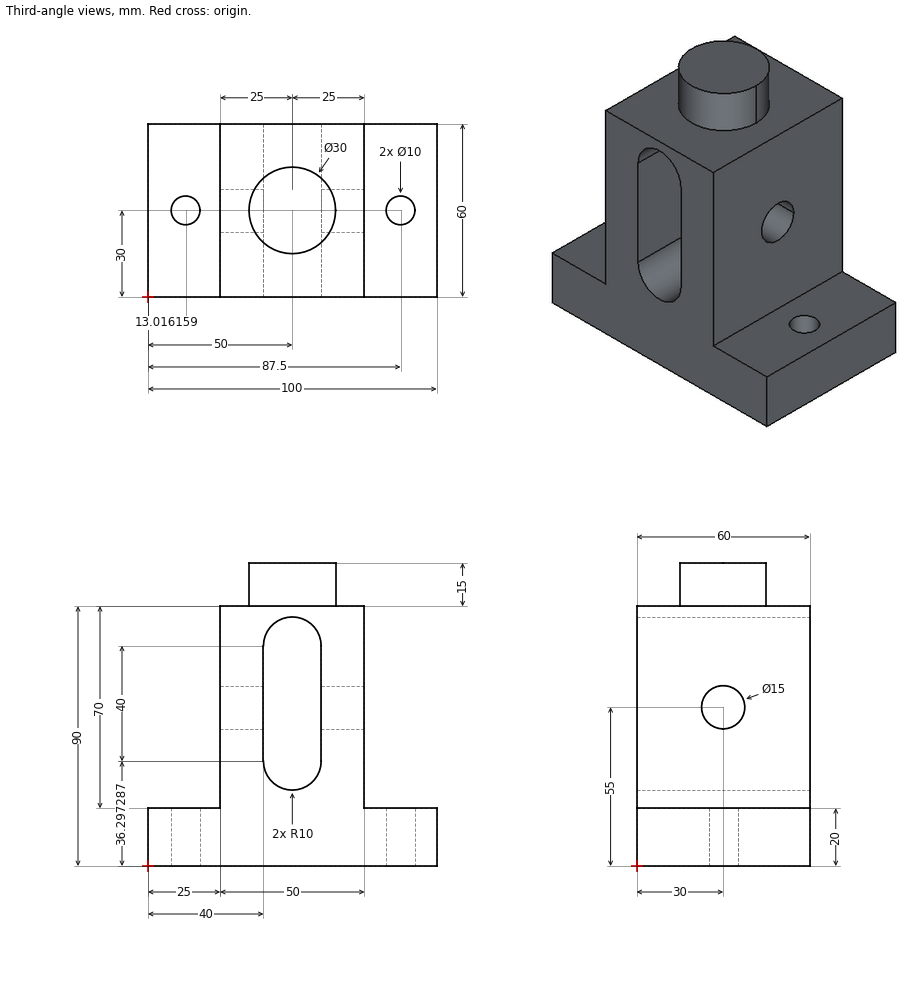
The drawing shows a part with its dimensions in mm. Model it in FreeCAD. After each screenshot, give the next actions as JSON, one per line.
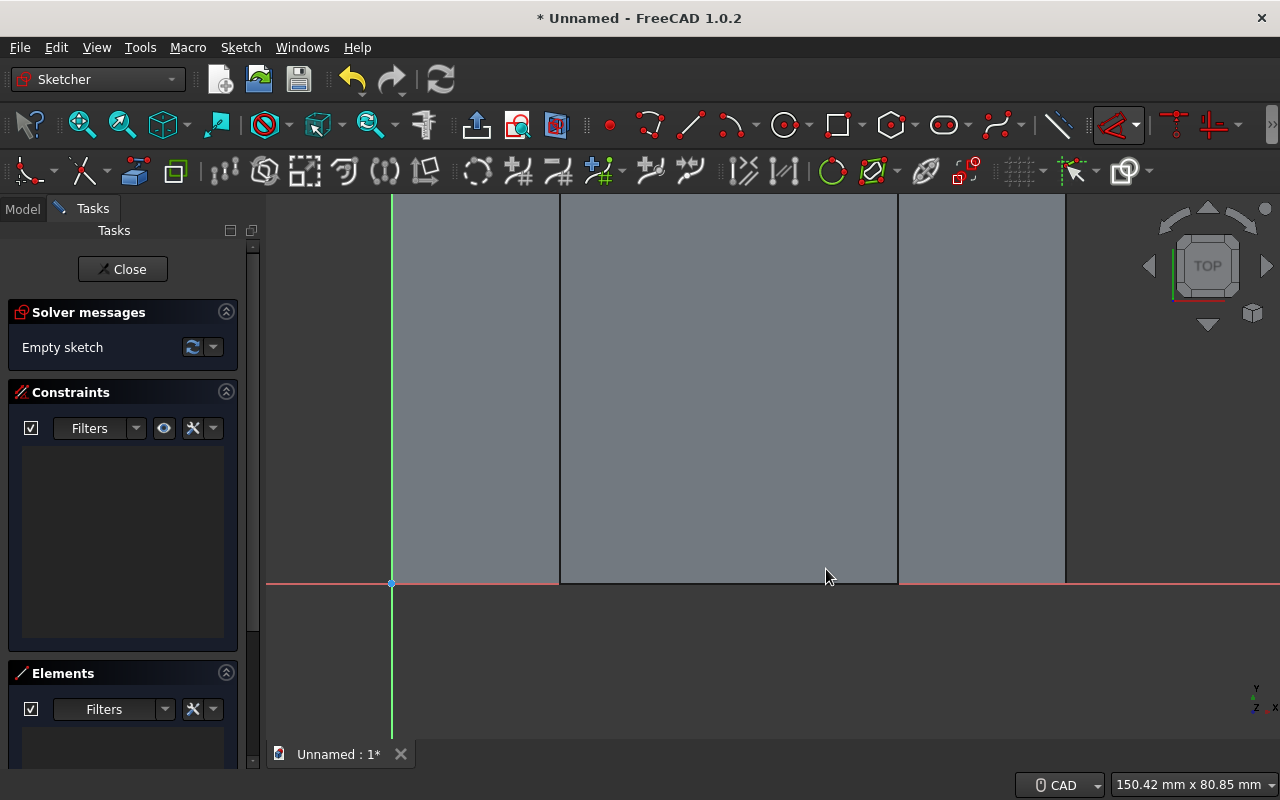
{"action": "left_click", "coordinate": [786, 126]}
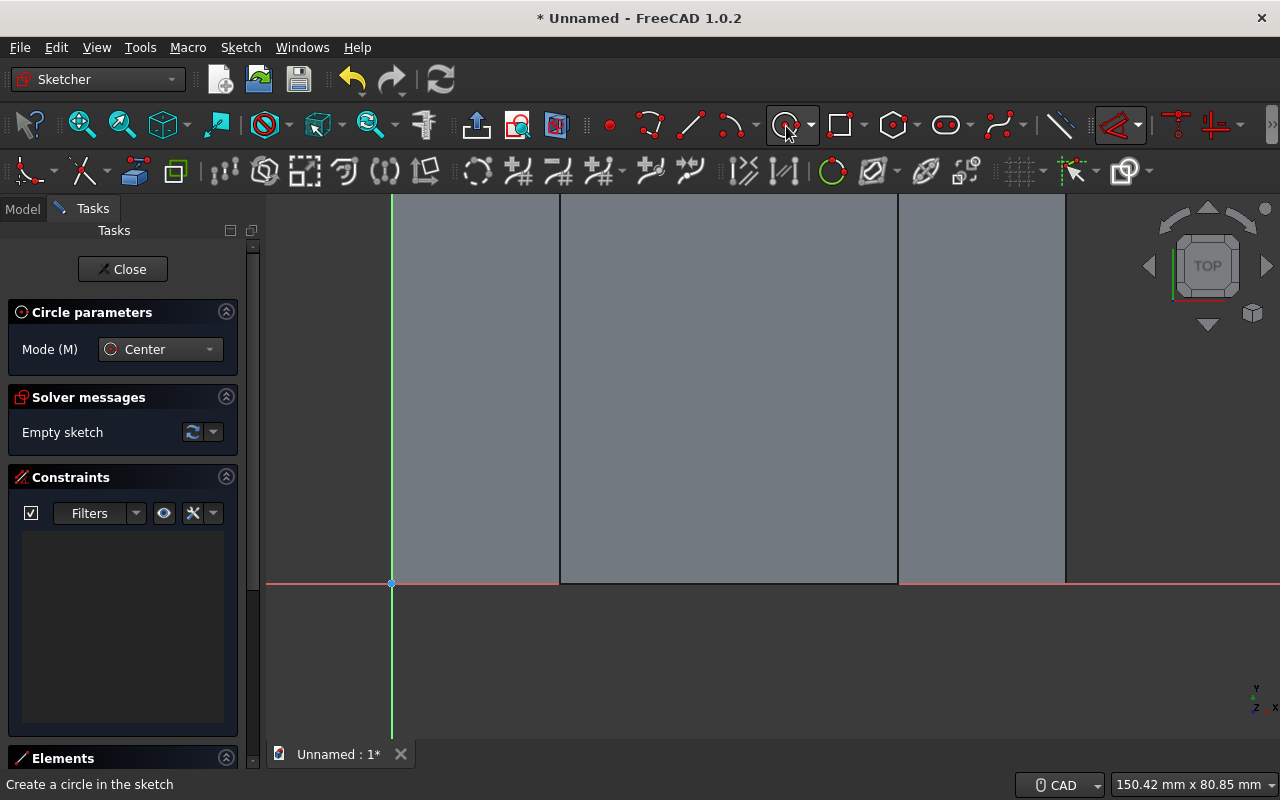
{"action": "left_click", "coordinate": [982, 382]}
{"action": "left_click", "coordinate": [1006, 358]}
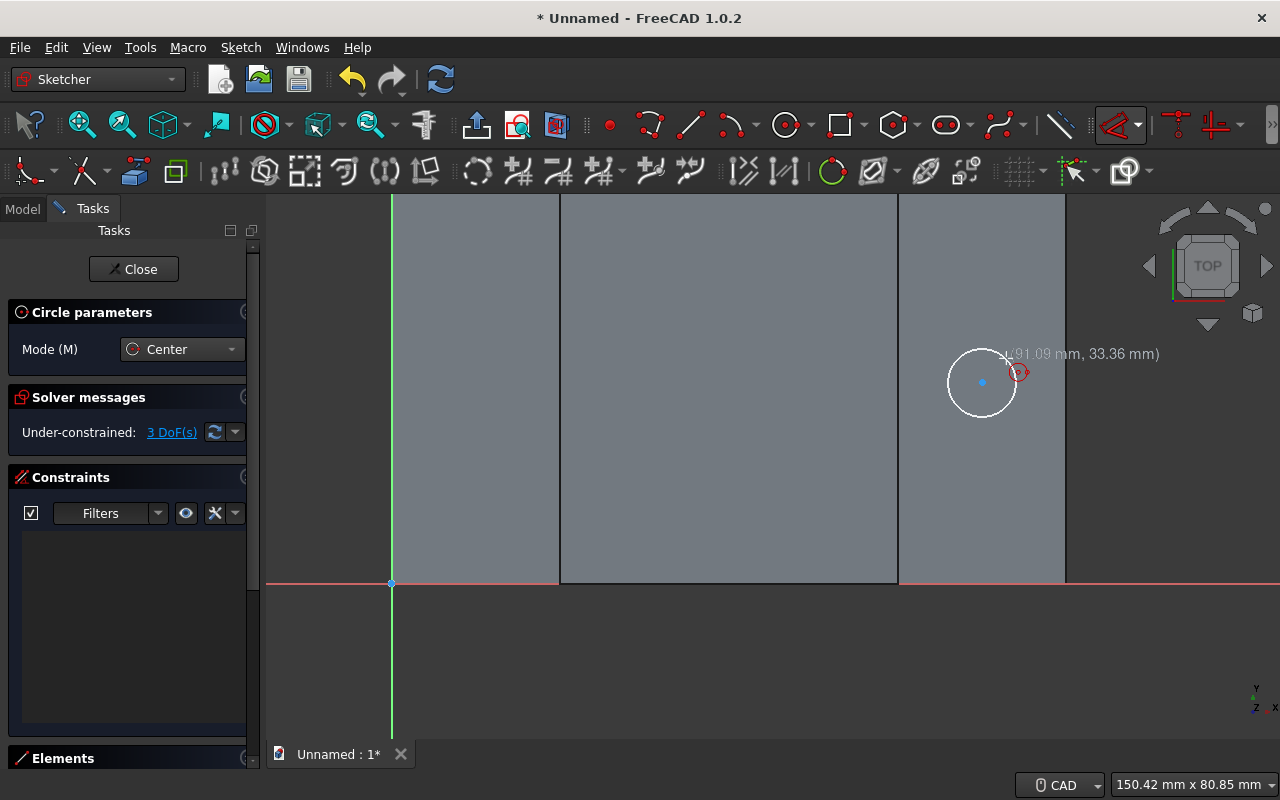
{"action": "left_click", "coordinate": [480, 382]}
{"action": "left_click", "coordinate": [503, 358]}
{"action": "key", "text": "Escape"}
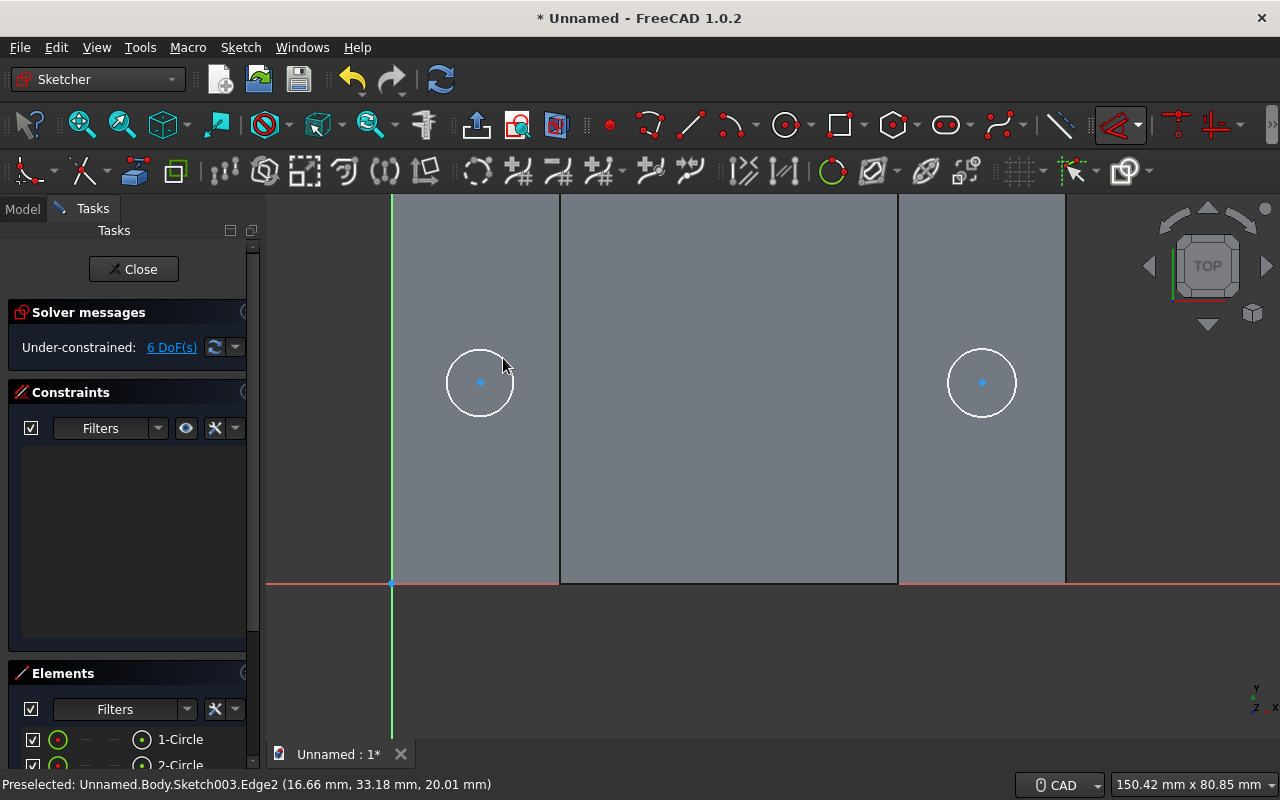
{"action": "left_click", "coordinate": [1006, 359]}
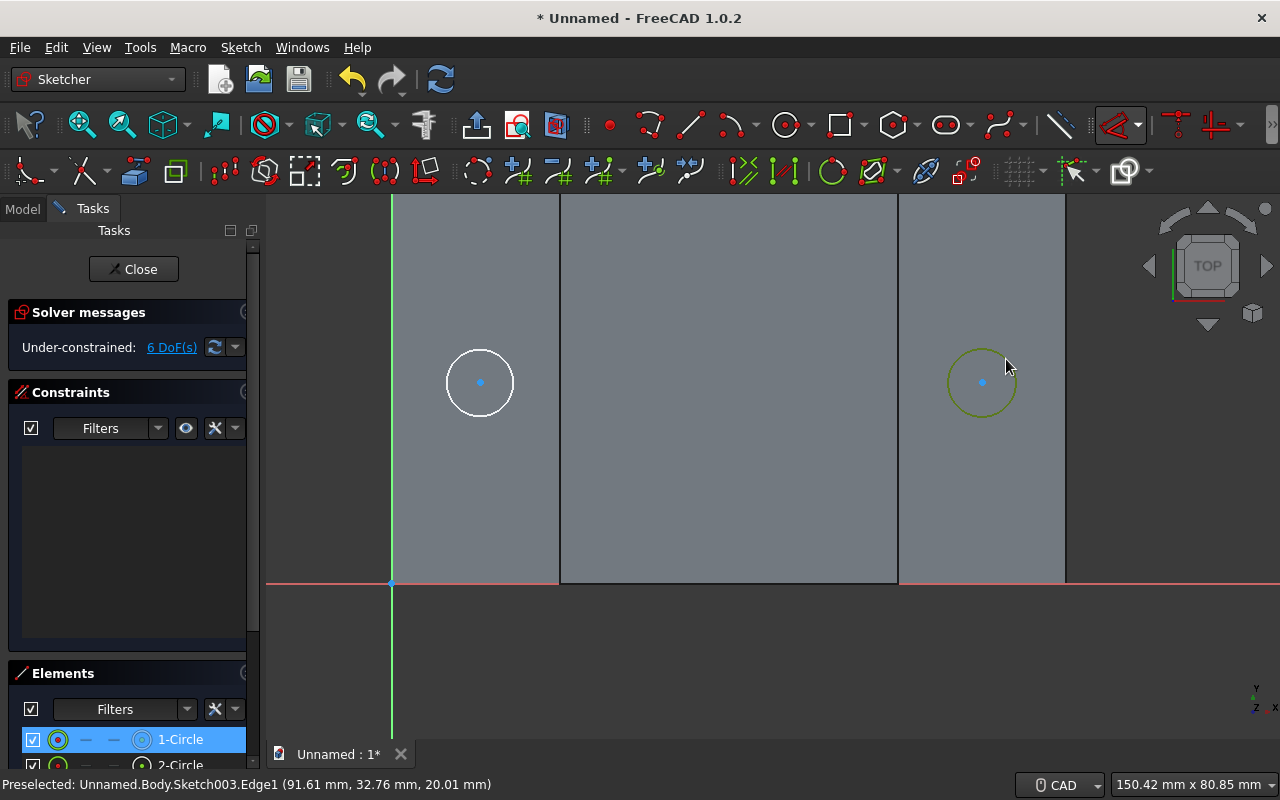
{"action": "left_click", "coordinate": [503, 359]}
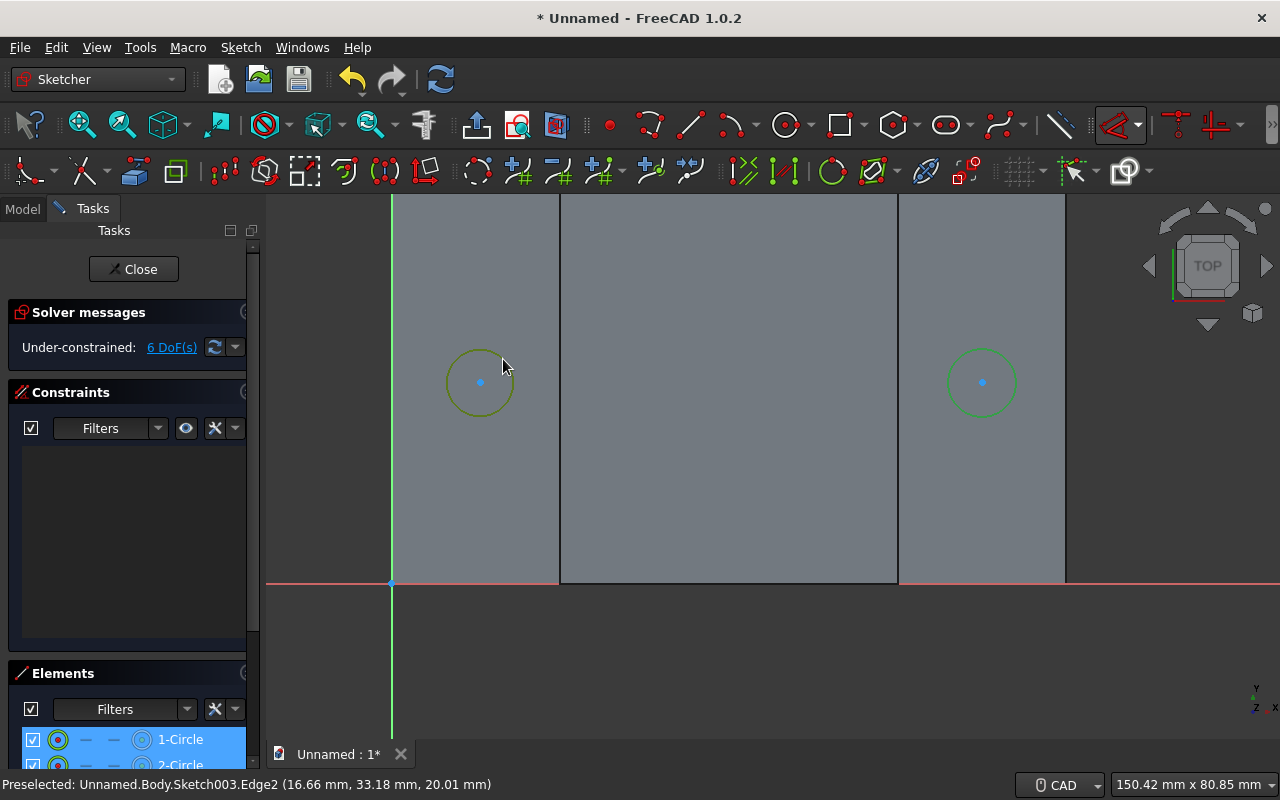
{"action": "key", "text": "e"}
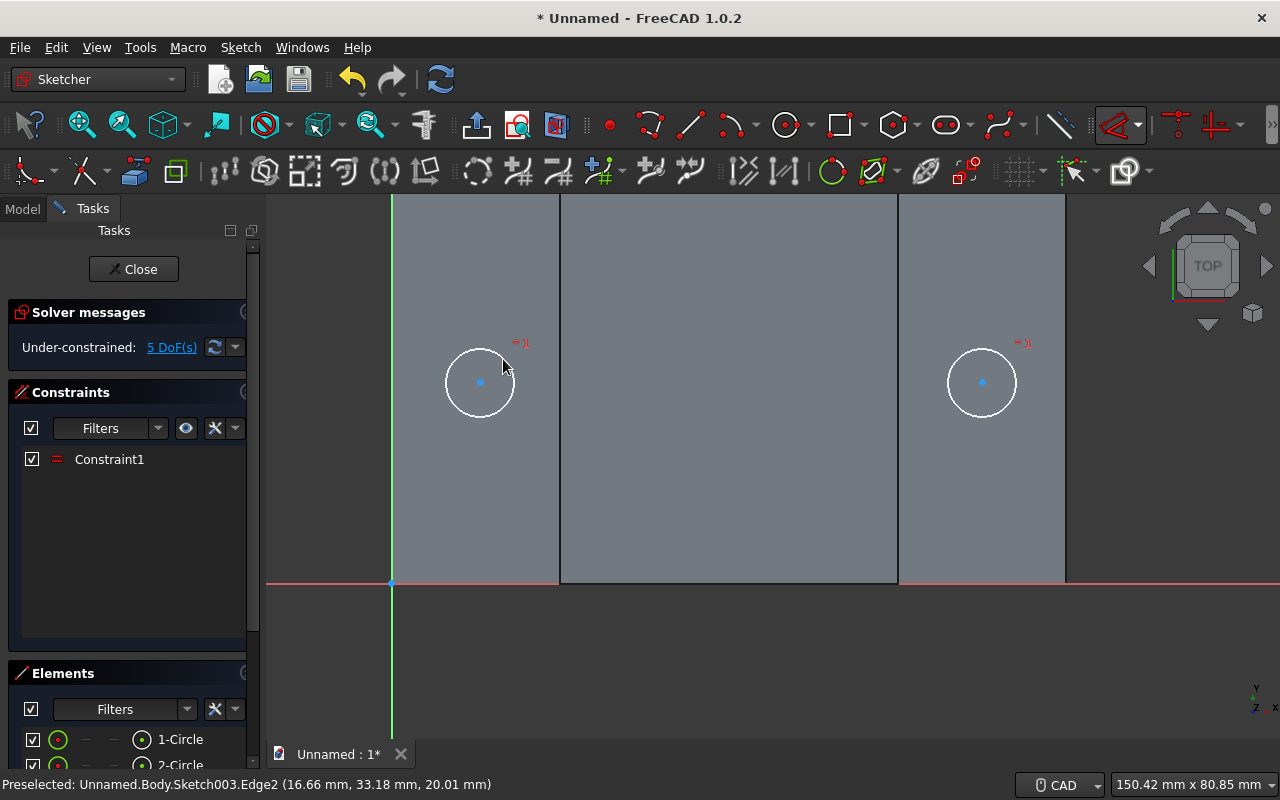
{"action": "left_click", "coordinate": [982, 383]}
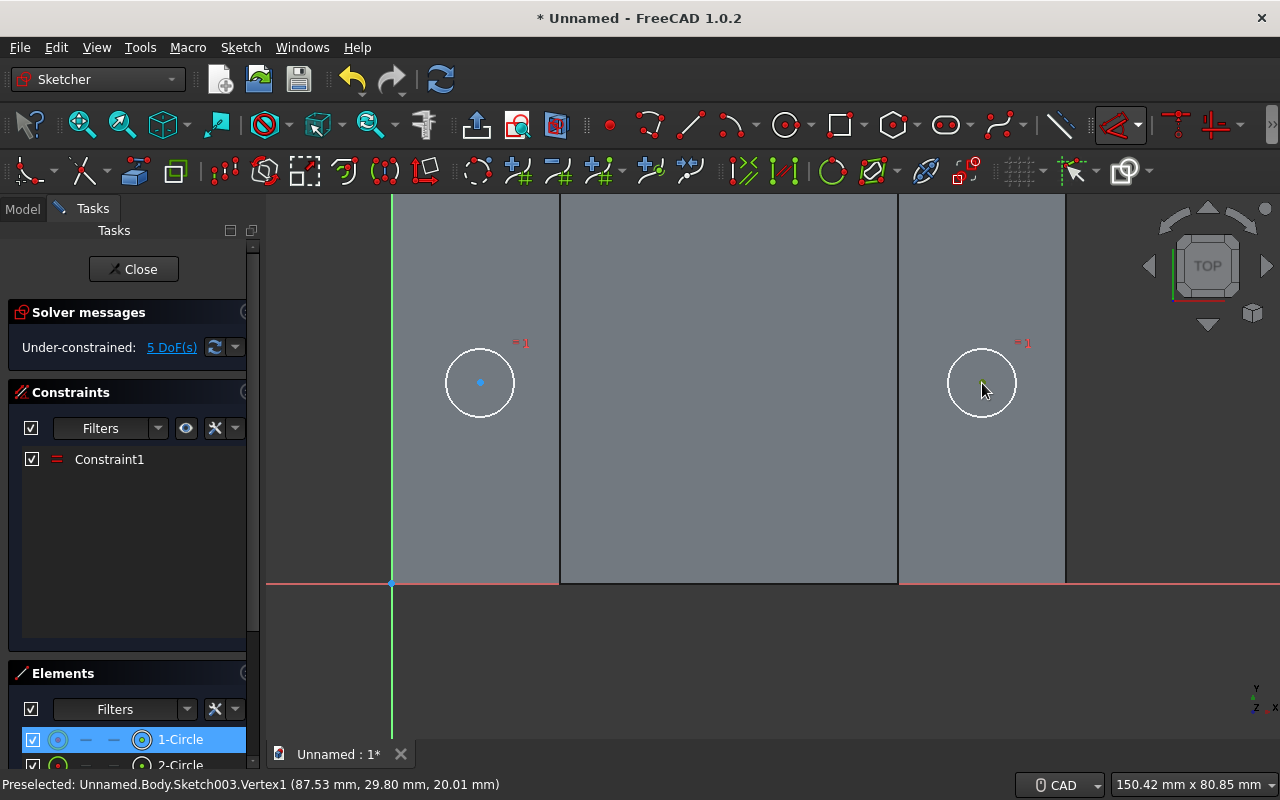
{"action": "left_click", "coordinate": [480, 383]}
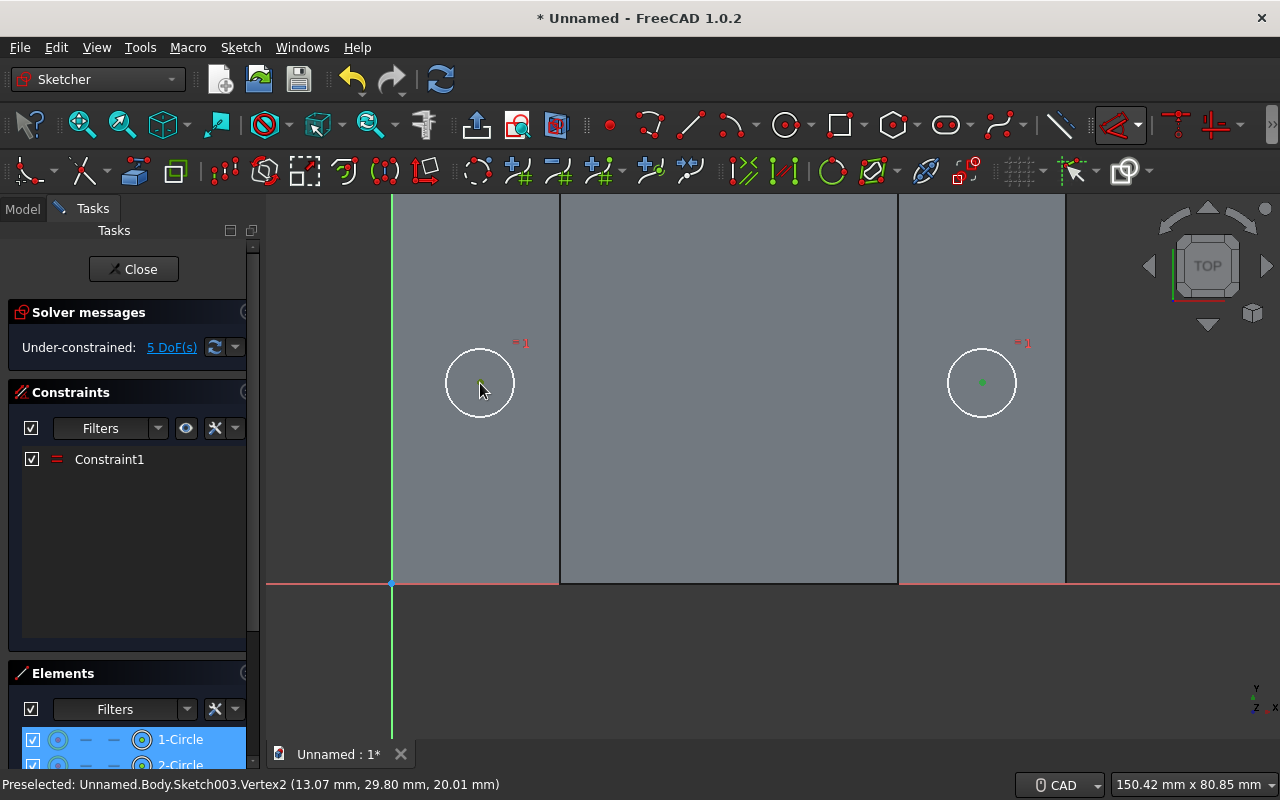
{"action": "key", "text": "h"}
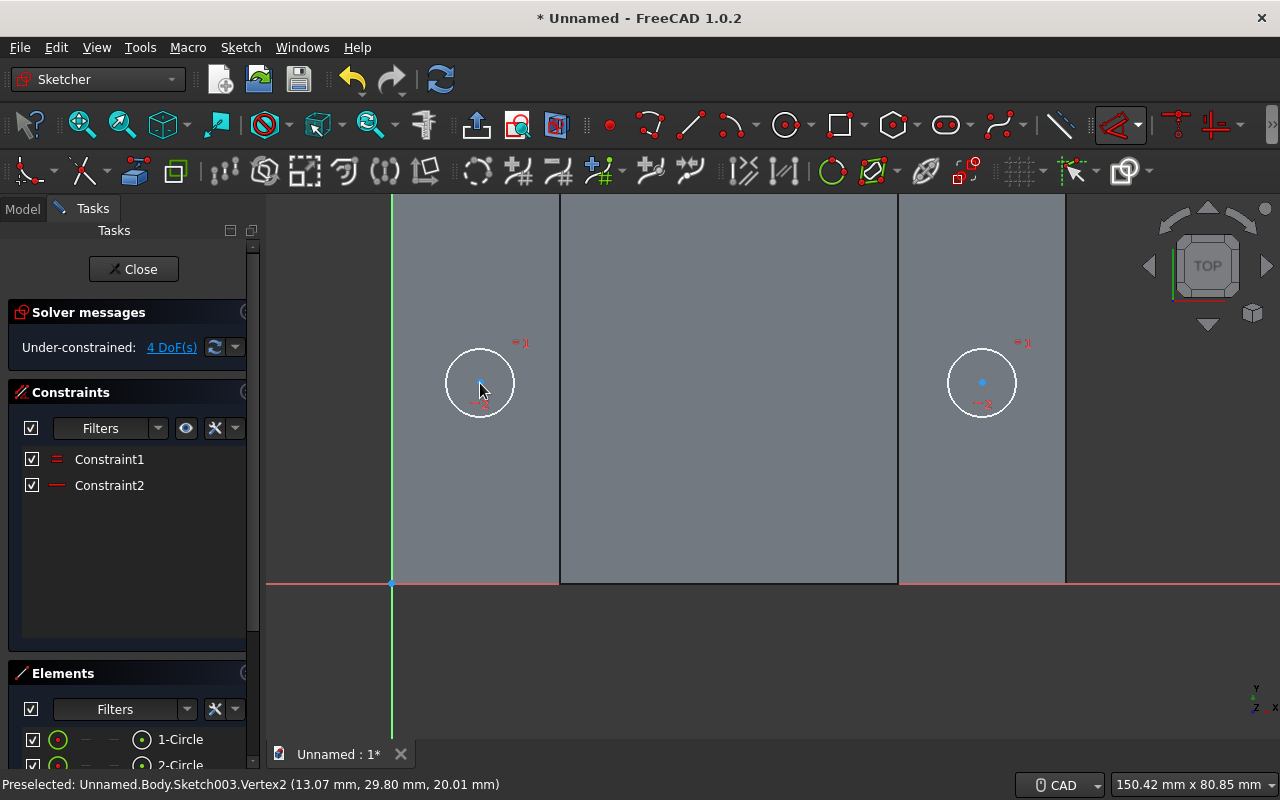
{"action": "left_click", "coordinate": [1006, 359]}